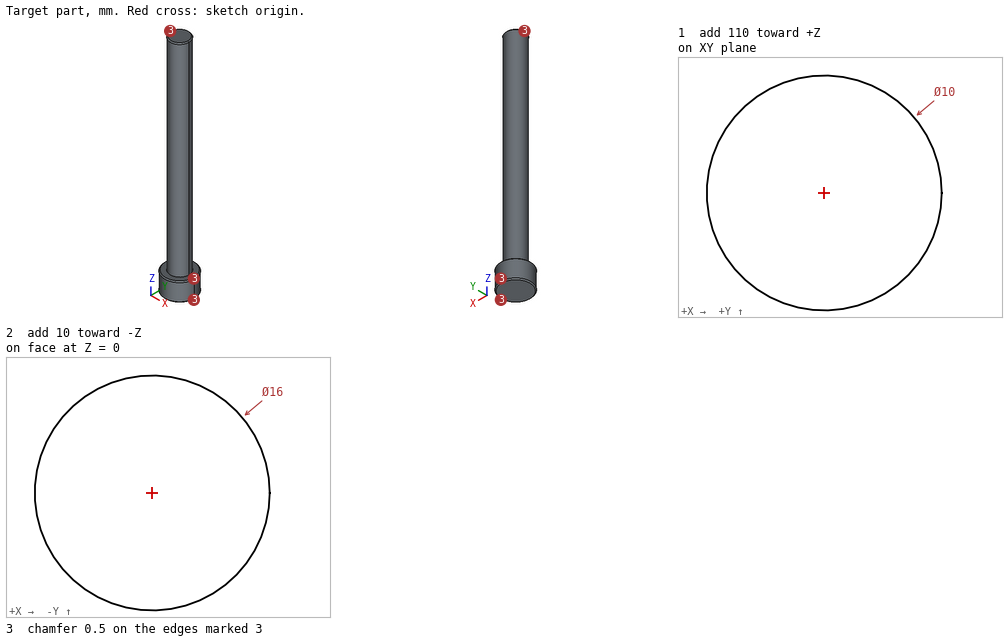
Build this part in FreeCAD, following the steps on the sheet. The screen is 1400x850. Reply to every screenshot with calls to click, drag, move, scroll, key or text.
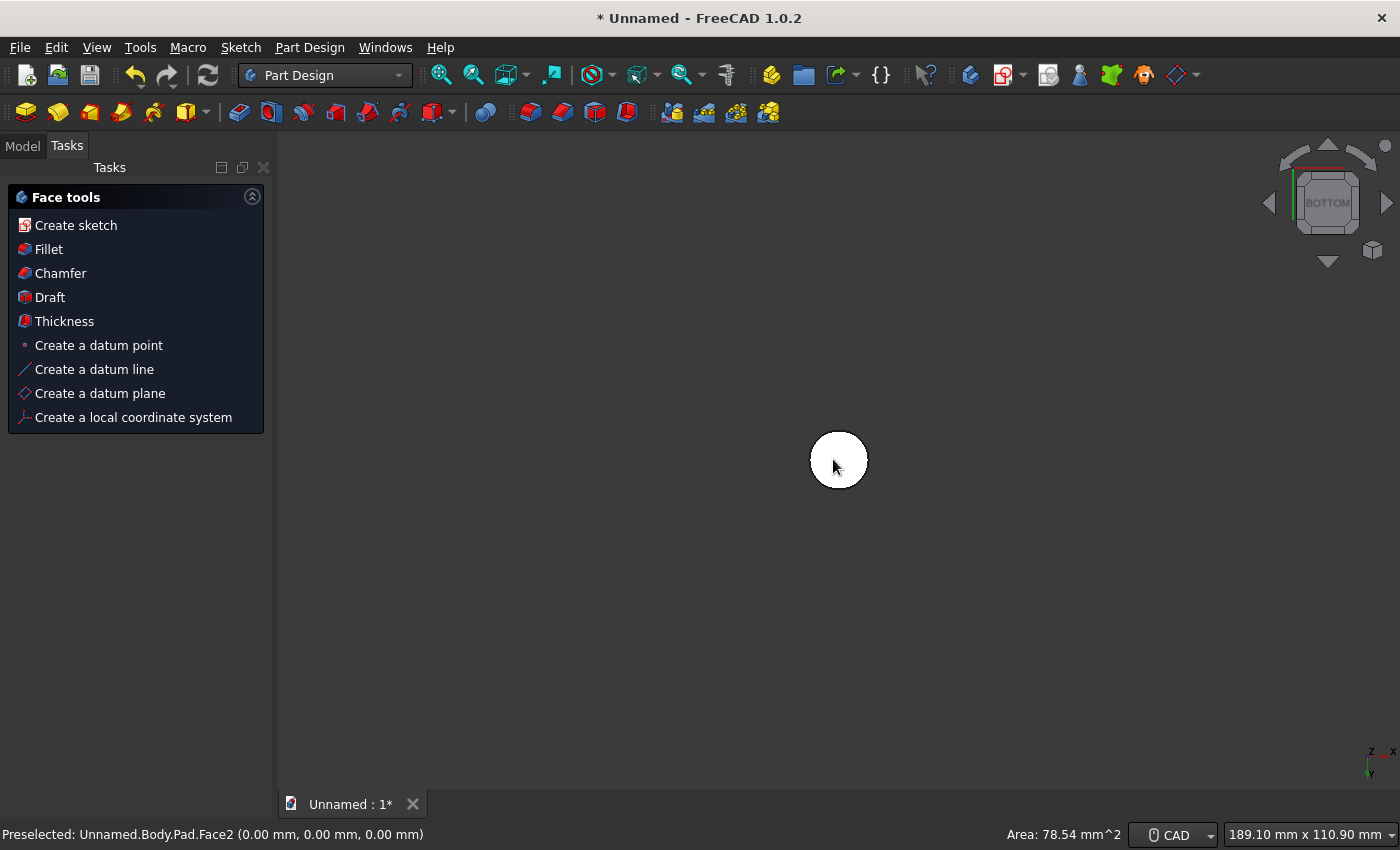
click(1004, 76)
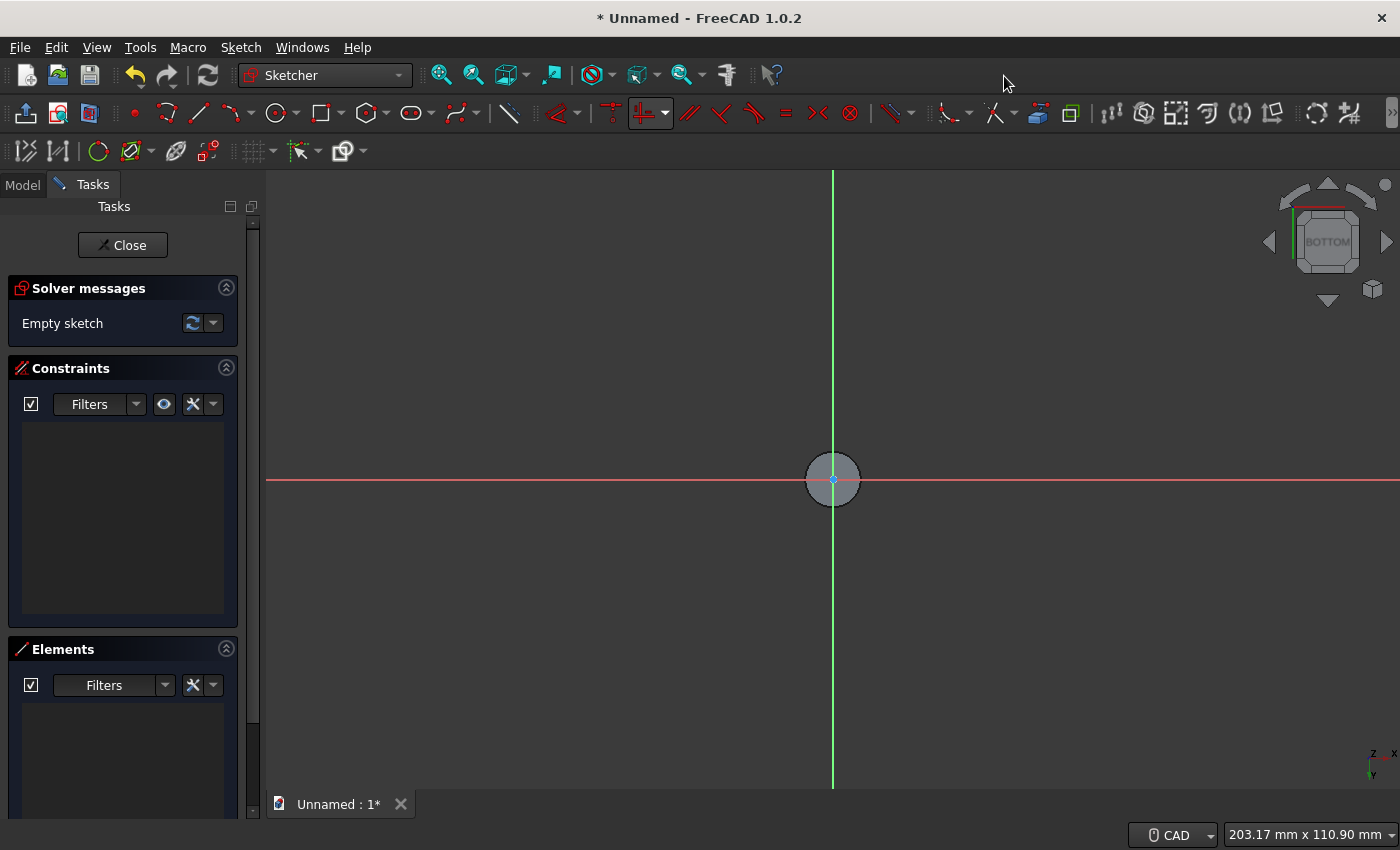
scroll(855, 480, up, 7)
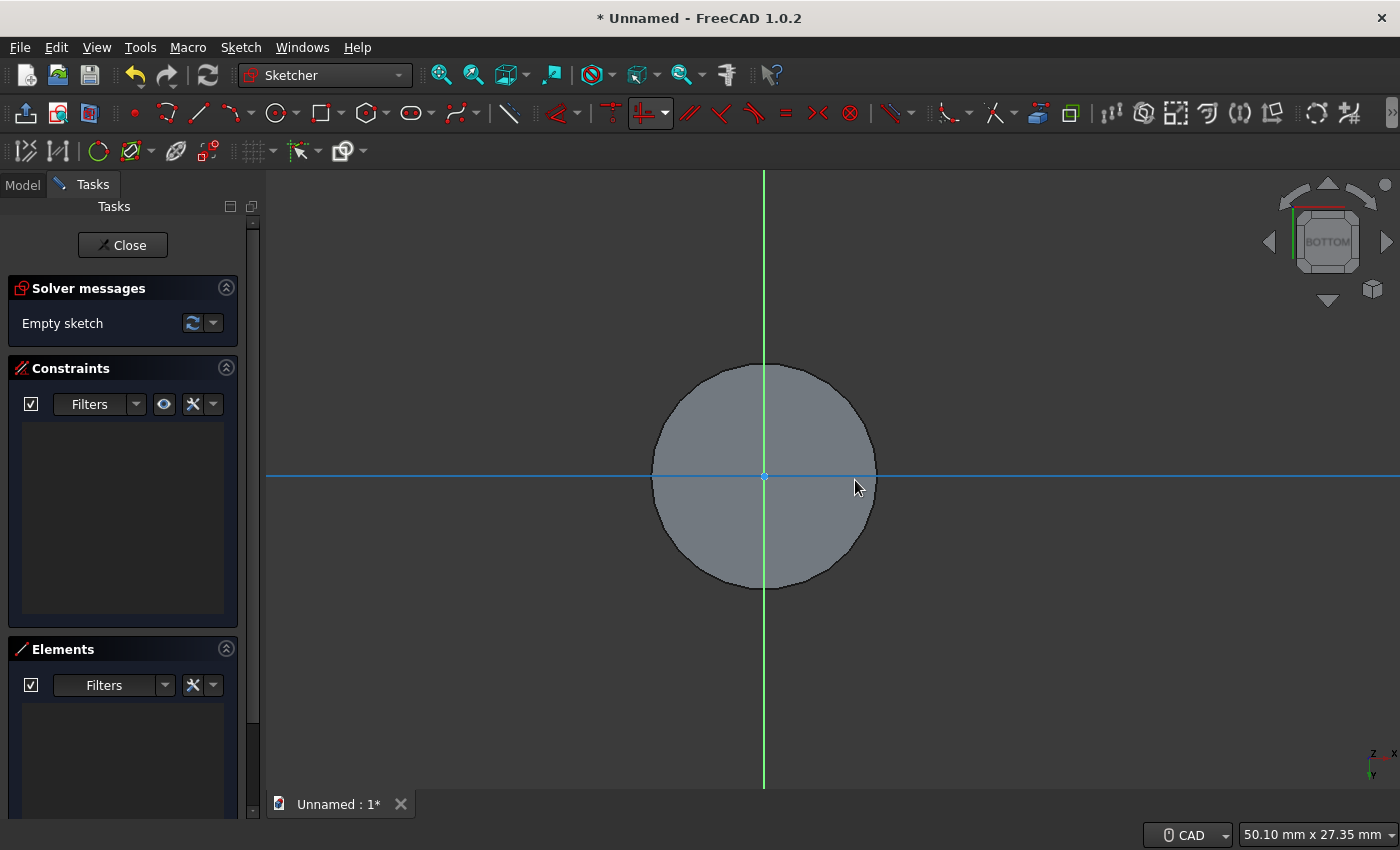
click(276, 114)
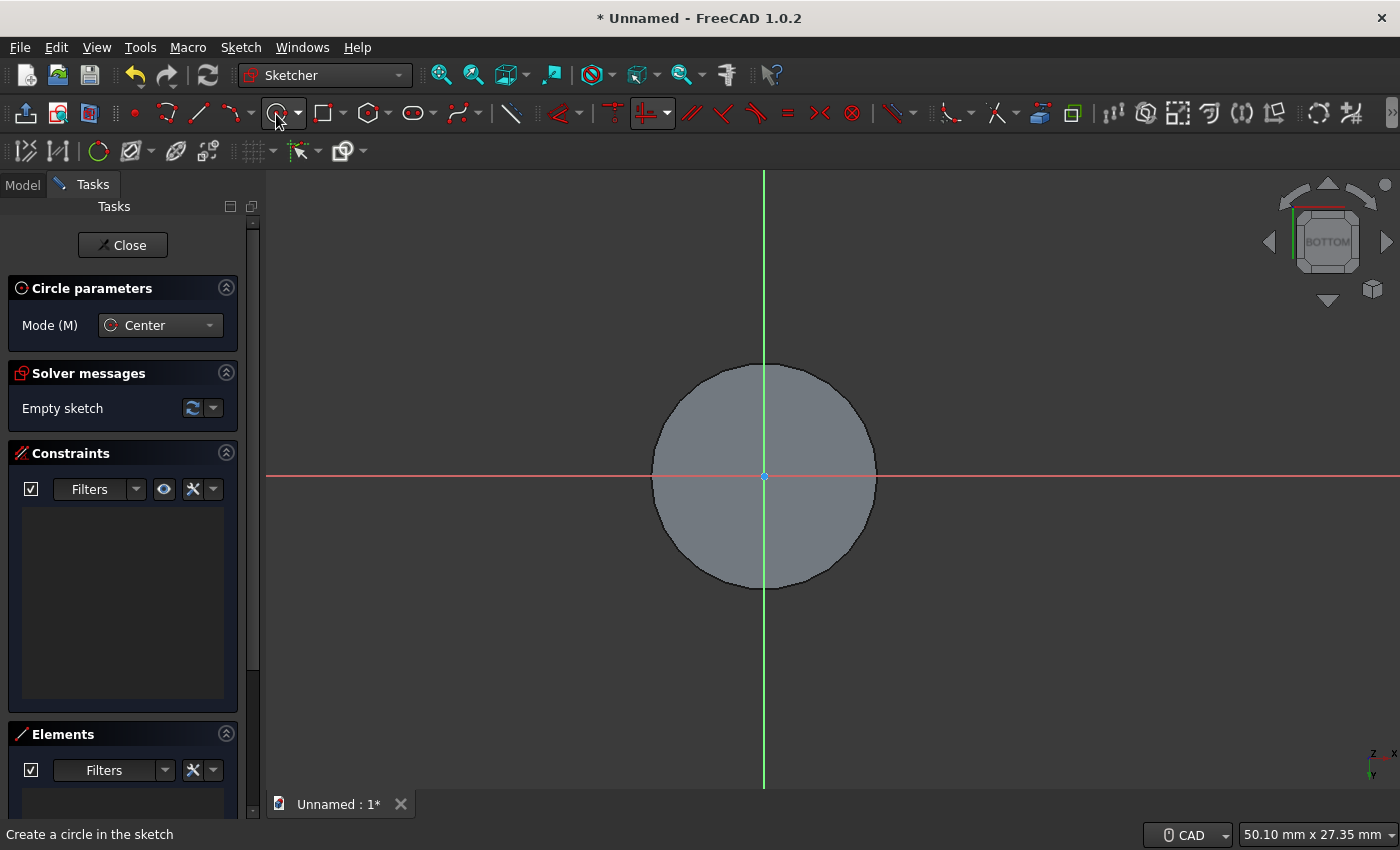
click(764, 476)
click(892, 348)
key(Escape)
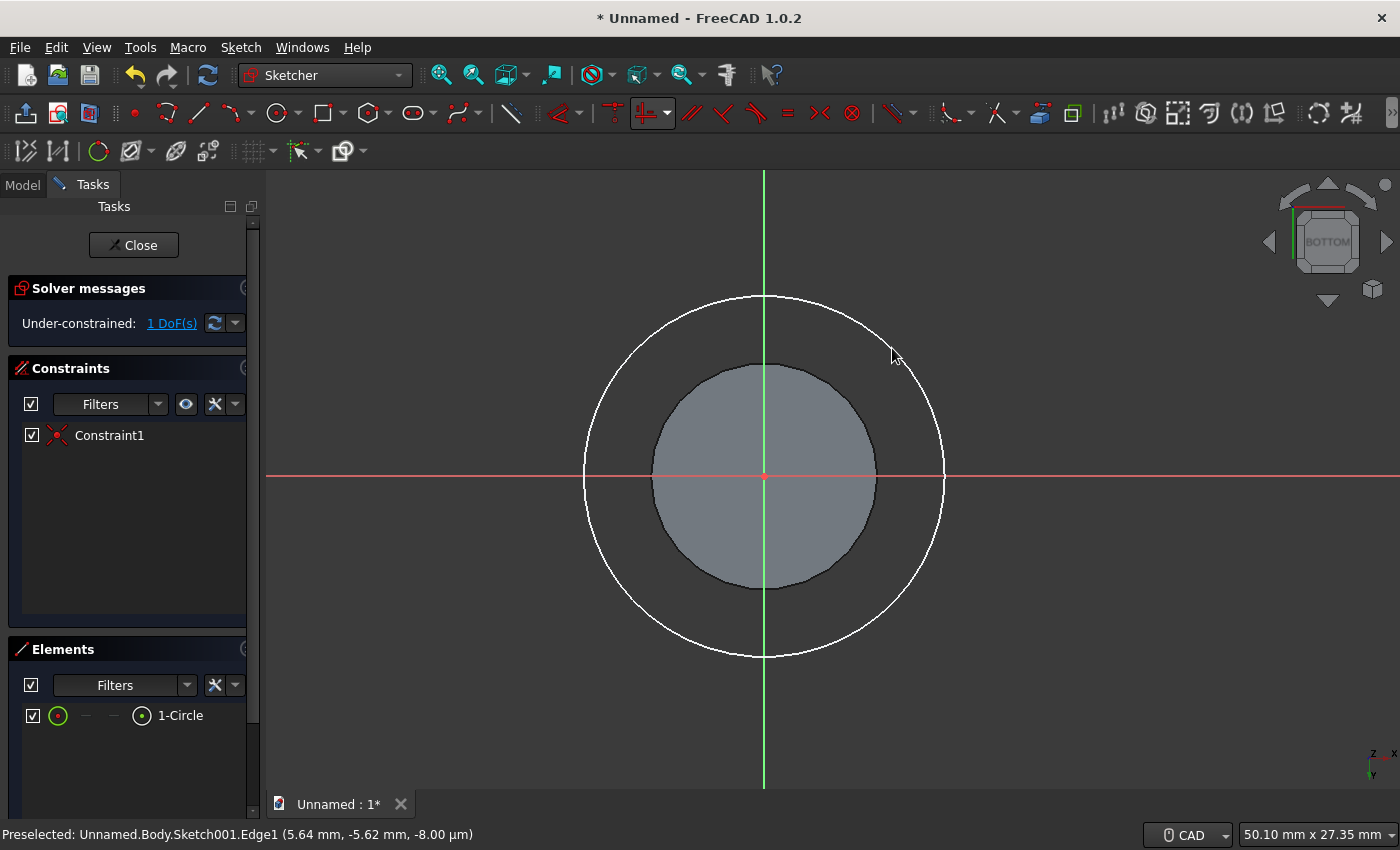
click(891, 348)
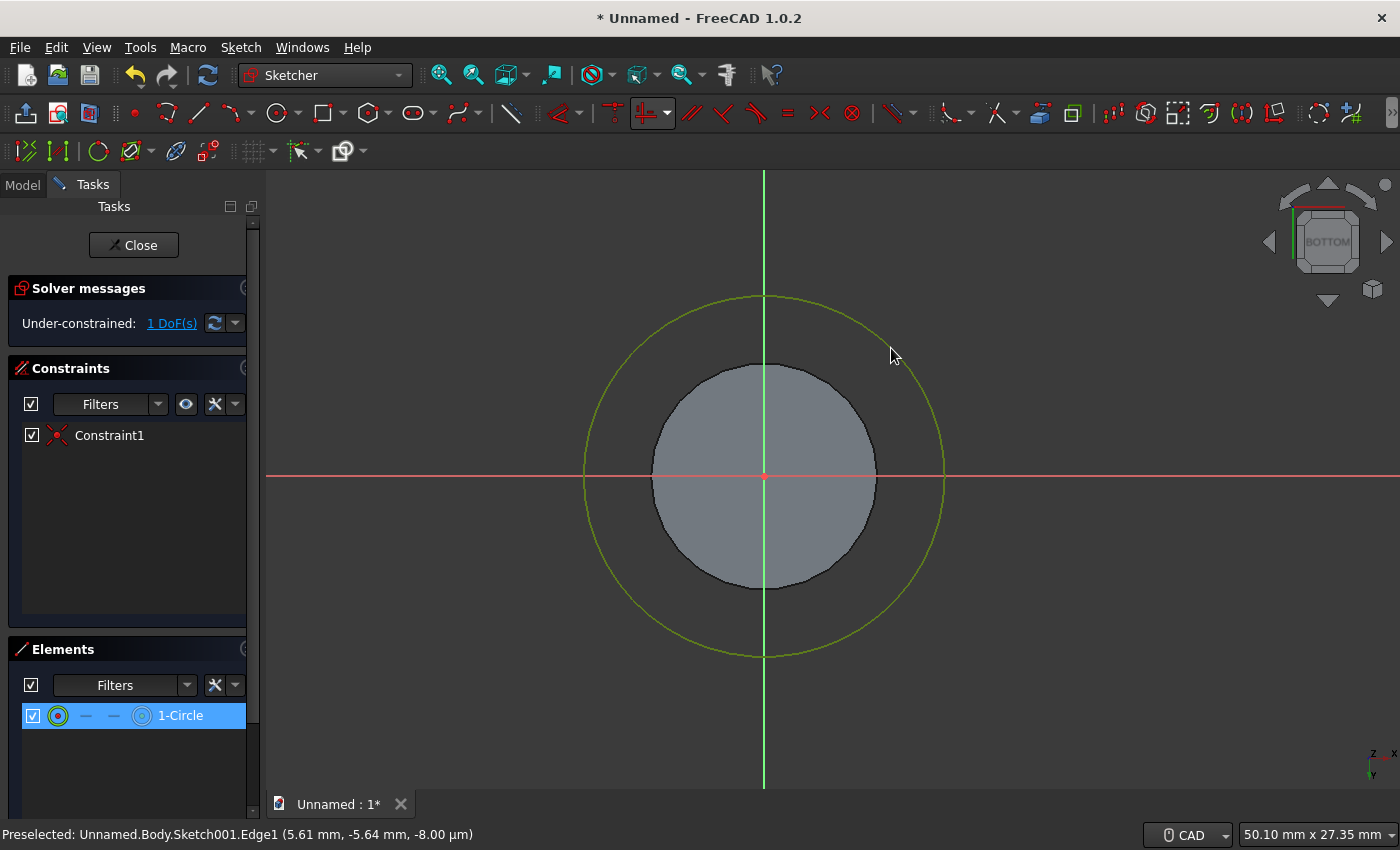
key(k)
key(o)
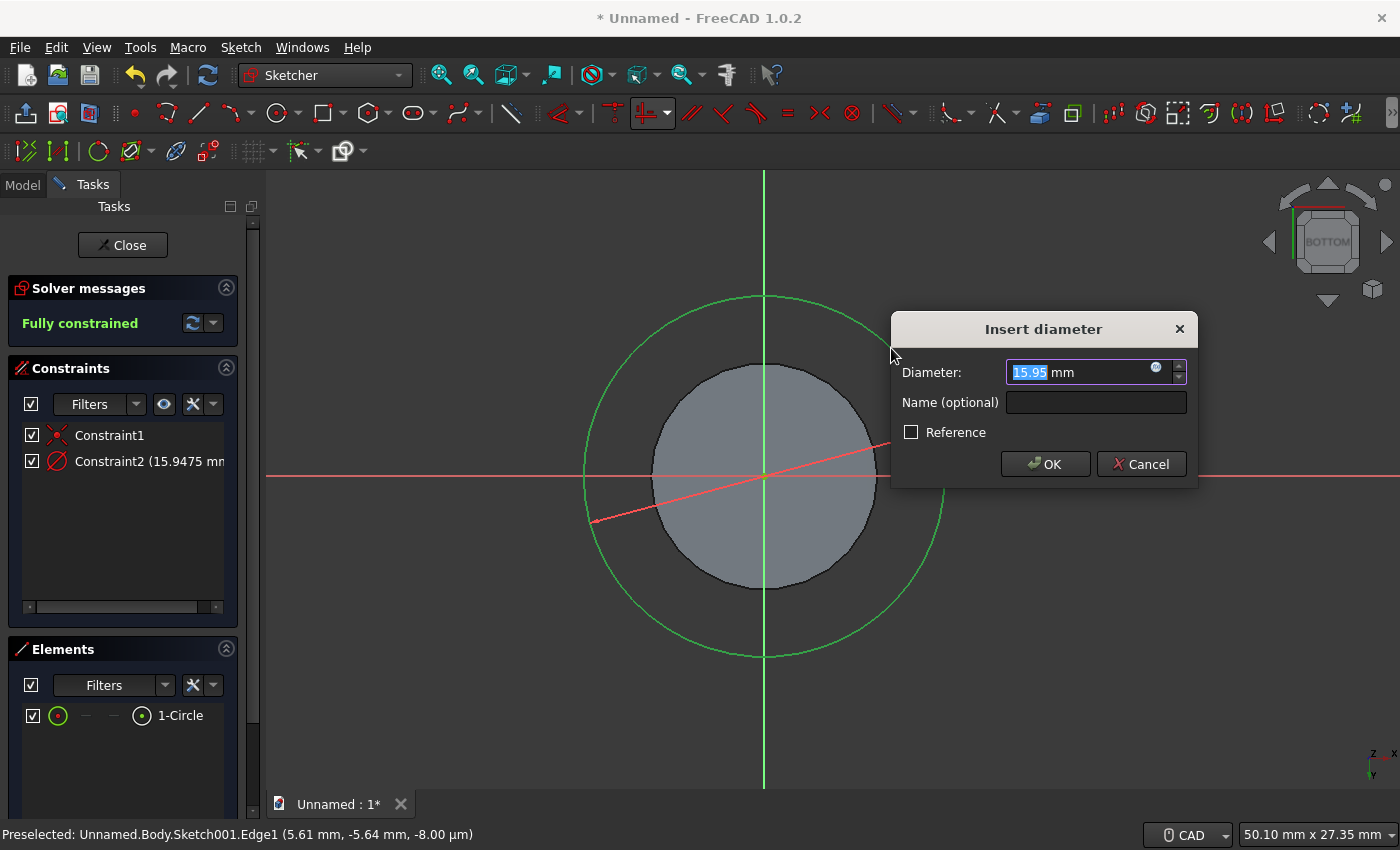
text(16)
key(Return)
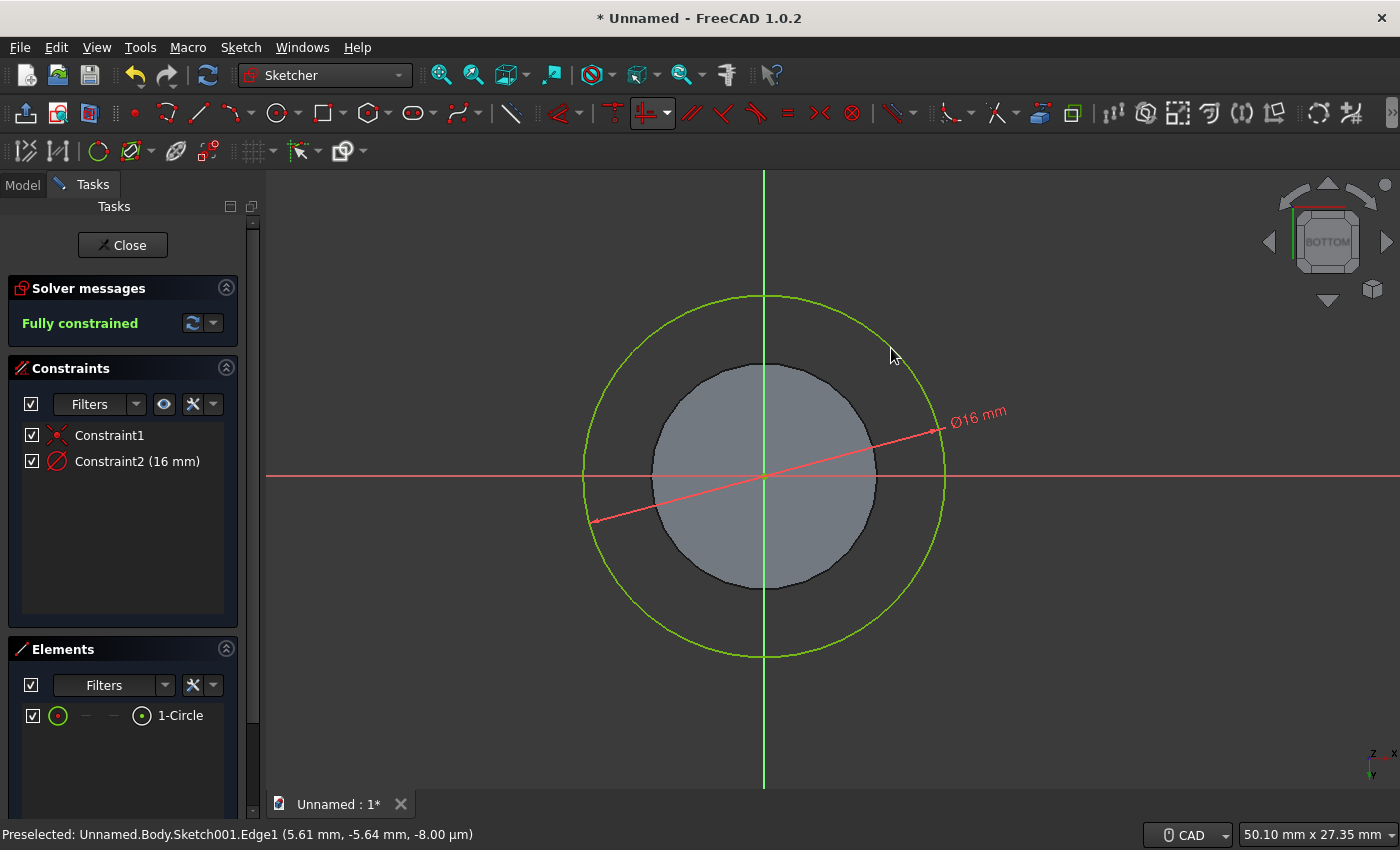
click(123, 245)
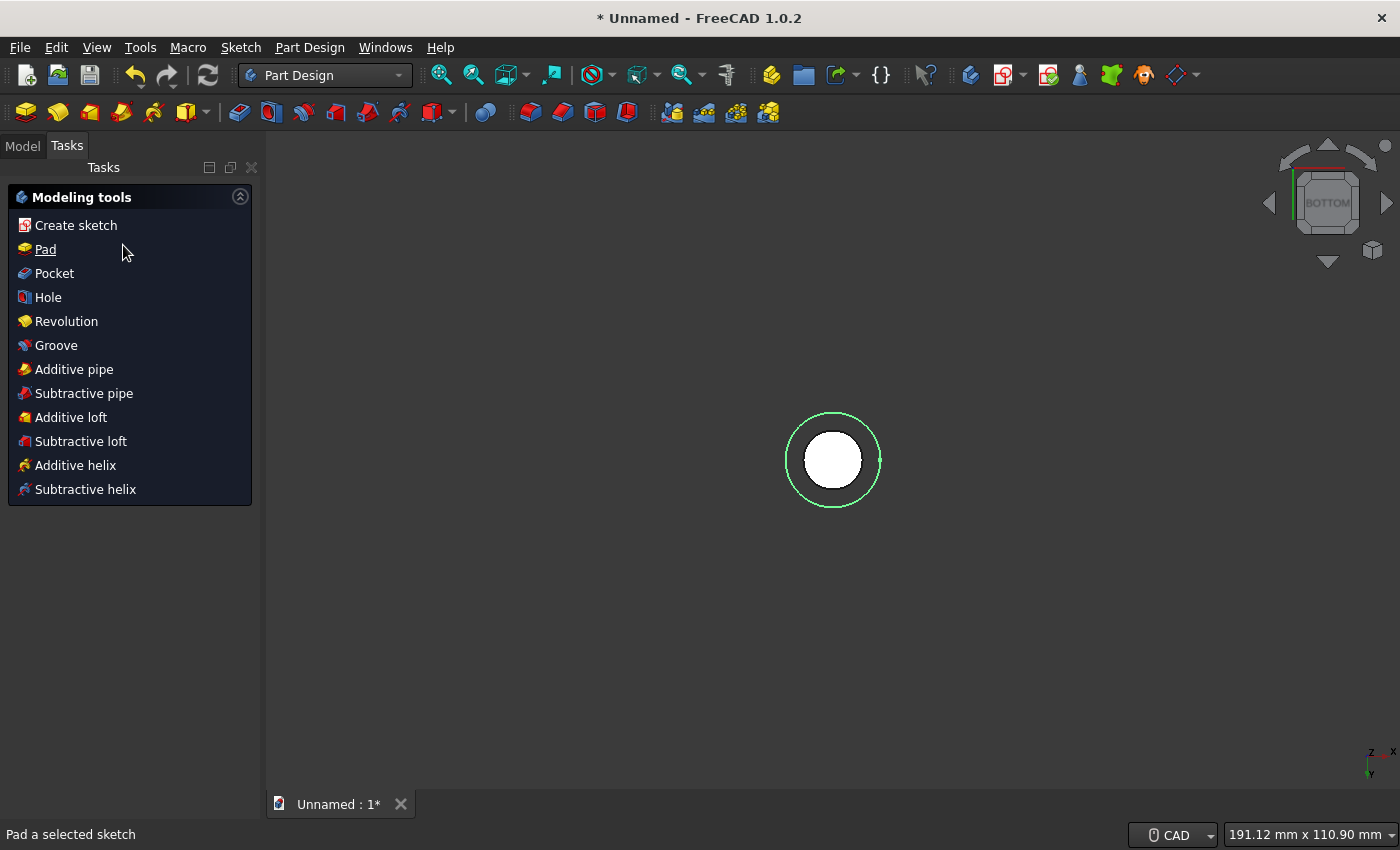
click(26, 112)